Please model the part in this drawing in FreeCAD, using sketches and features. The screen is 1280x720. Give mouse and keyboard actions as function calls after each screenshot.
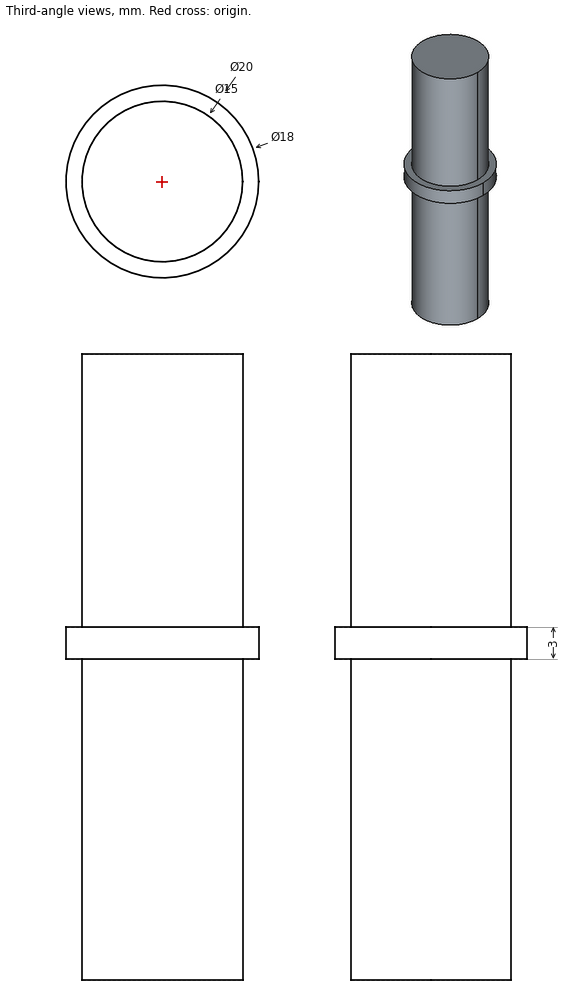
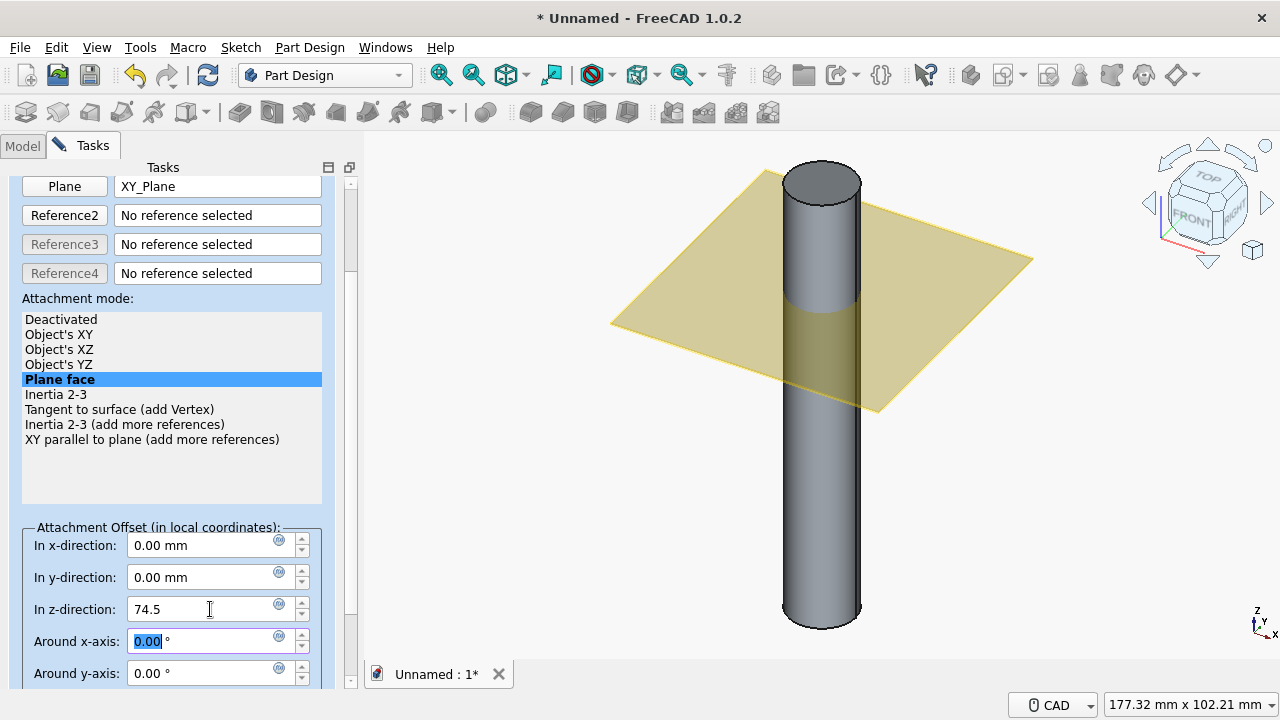
scroll(351, 432, up, 3)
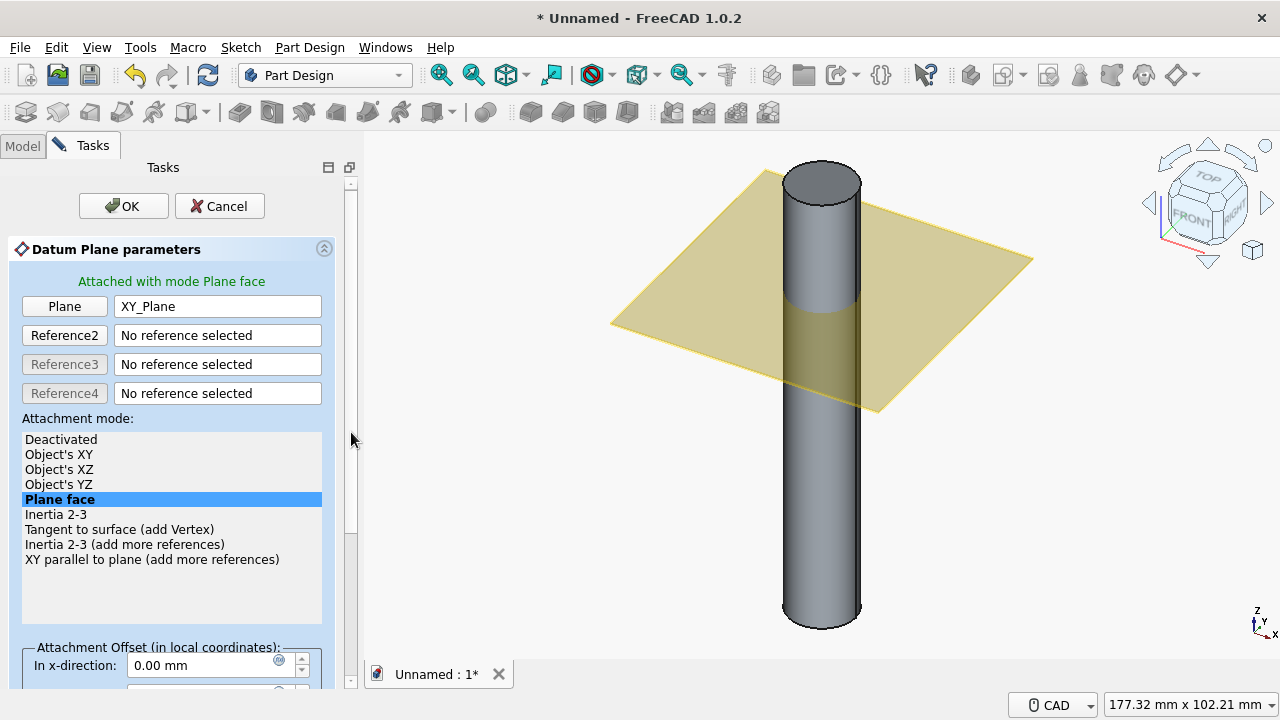
click(124, 206)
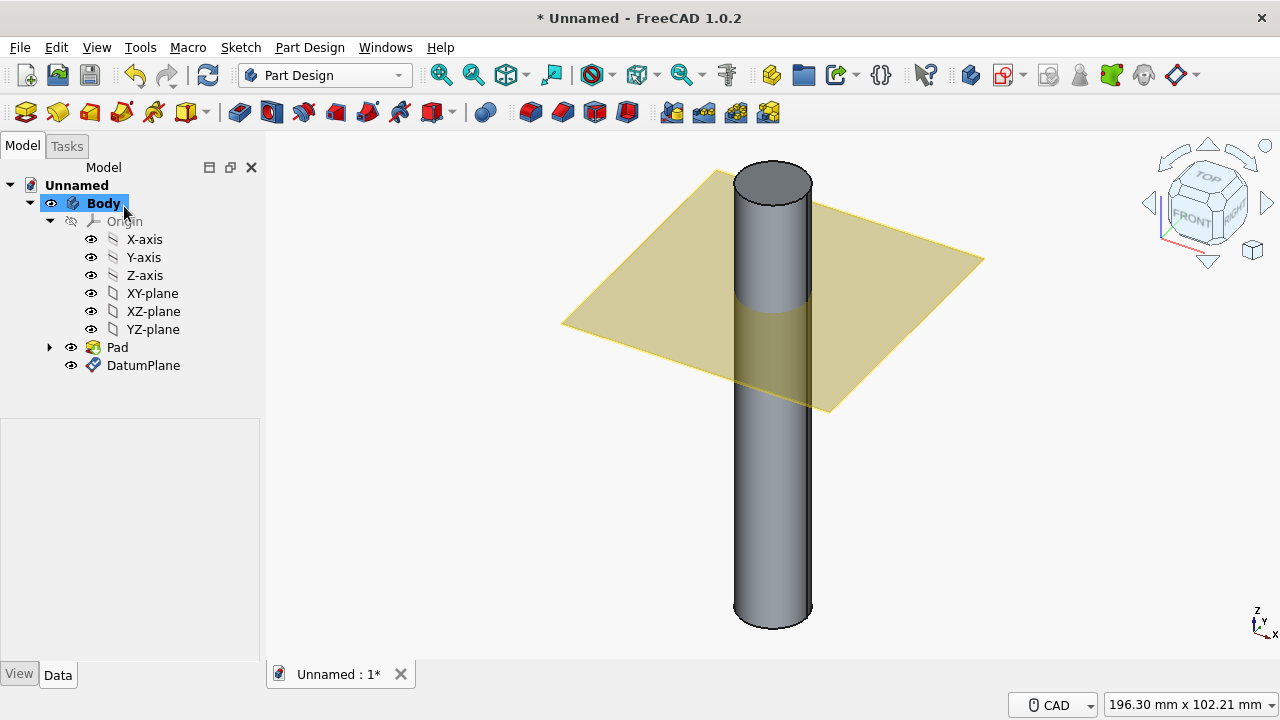
click(116, 365)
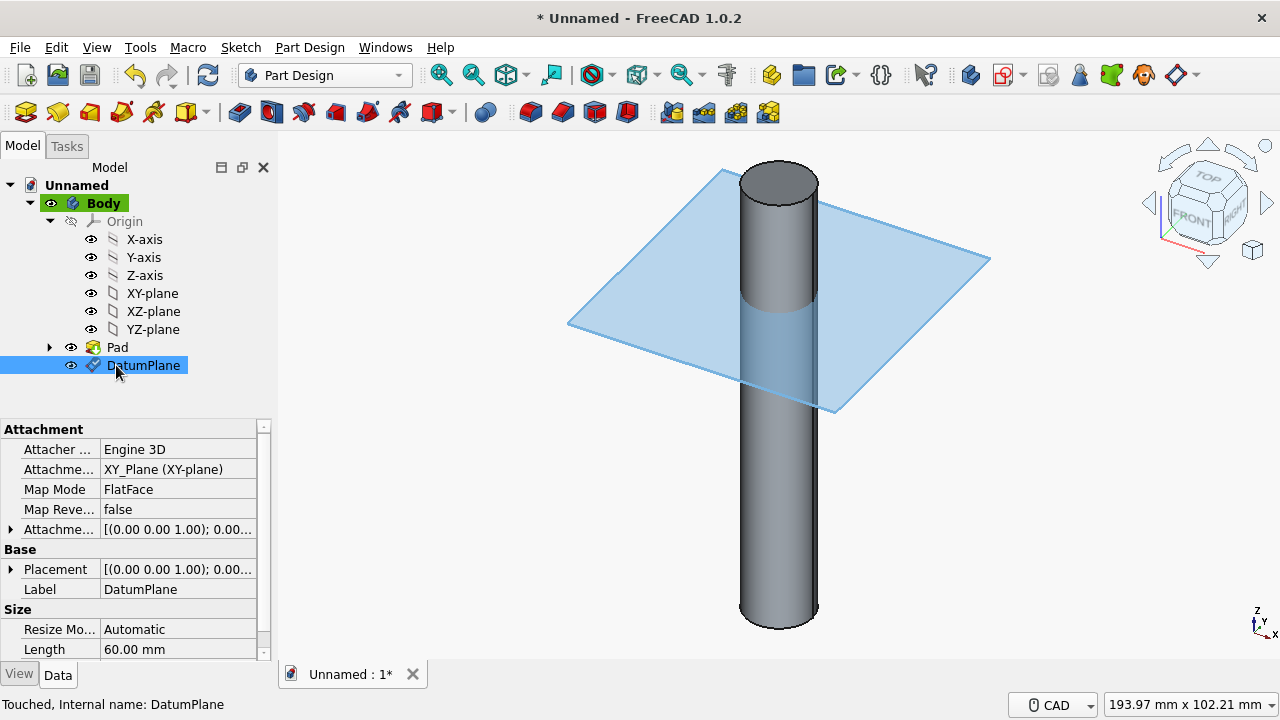
click(1004, 76)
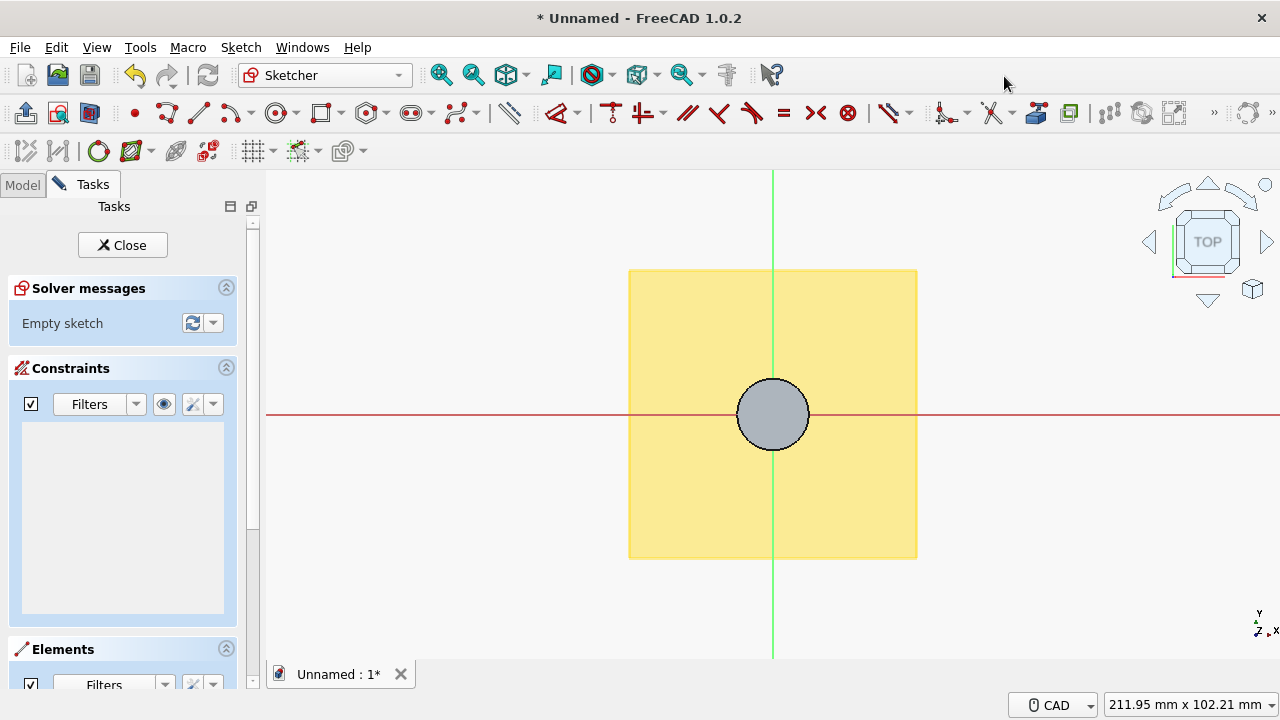
click(90, 114)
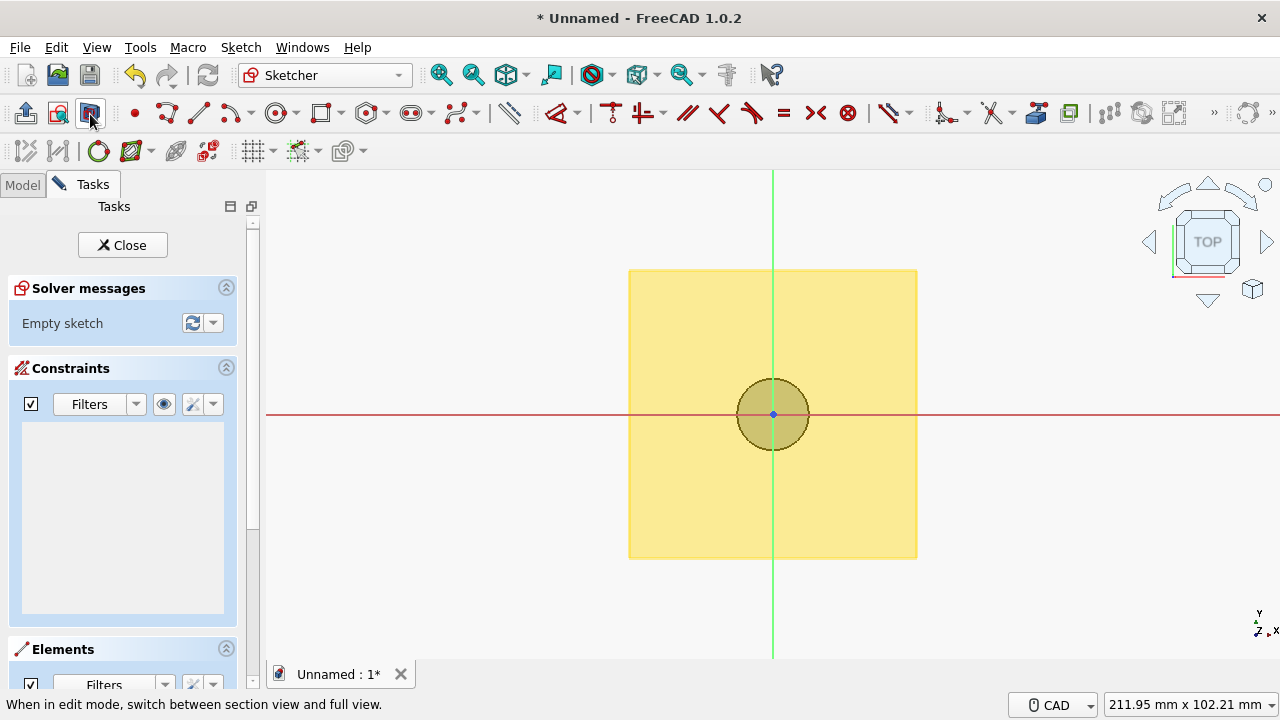
scroll(803, 415, up, 6)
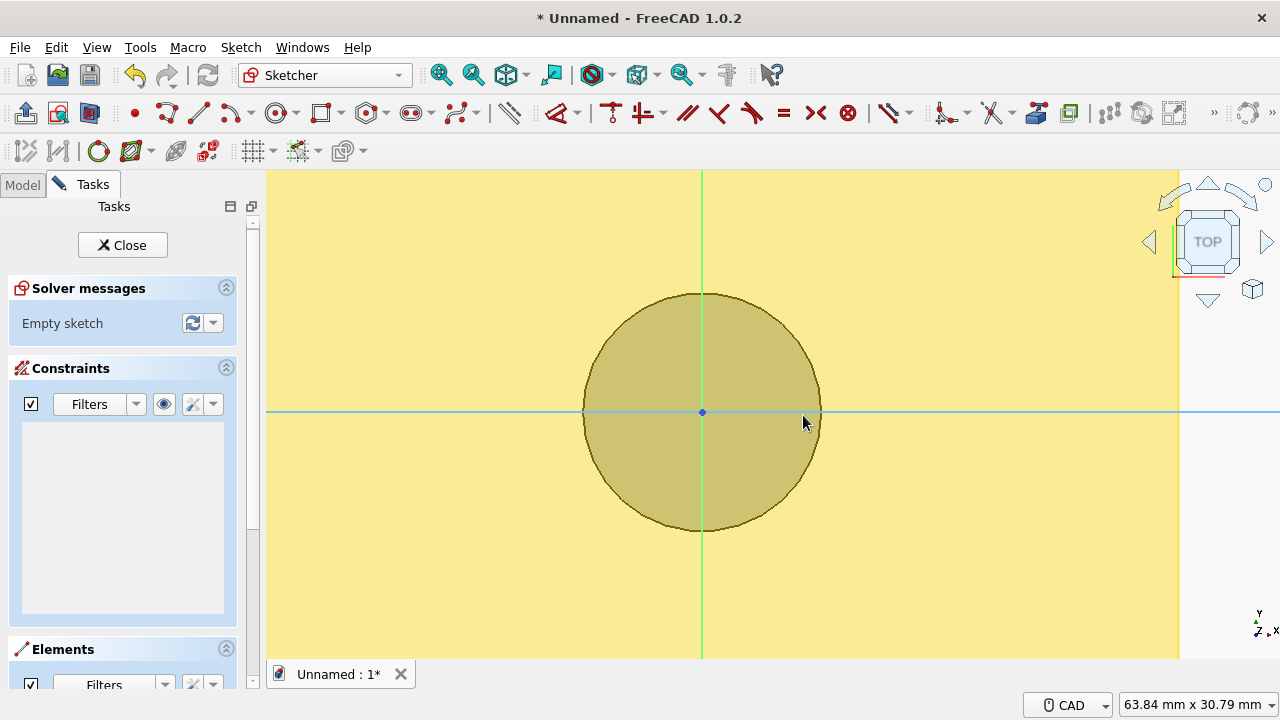
click(276, 114)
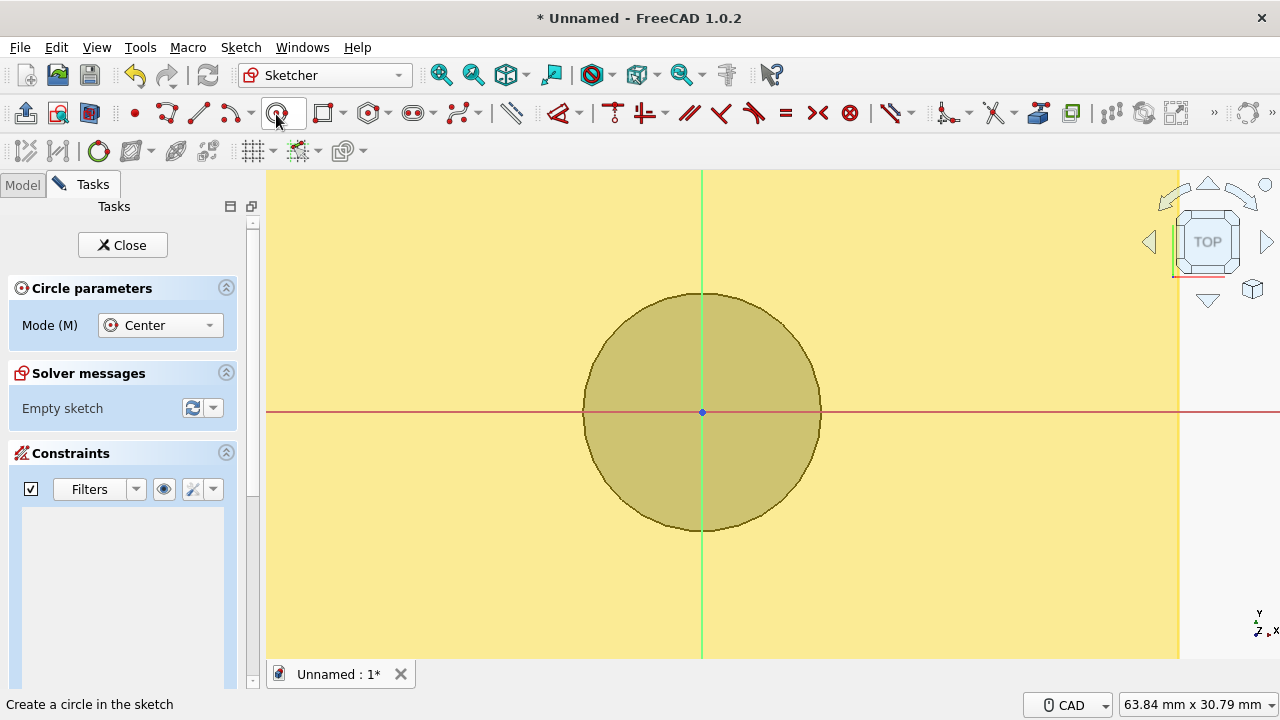
click(702, 412)
click(803, 311)
key(Escape)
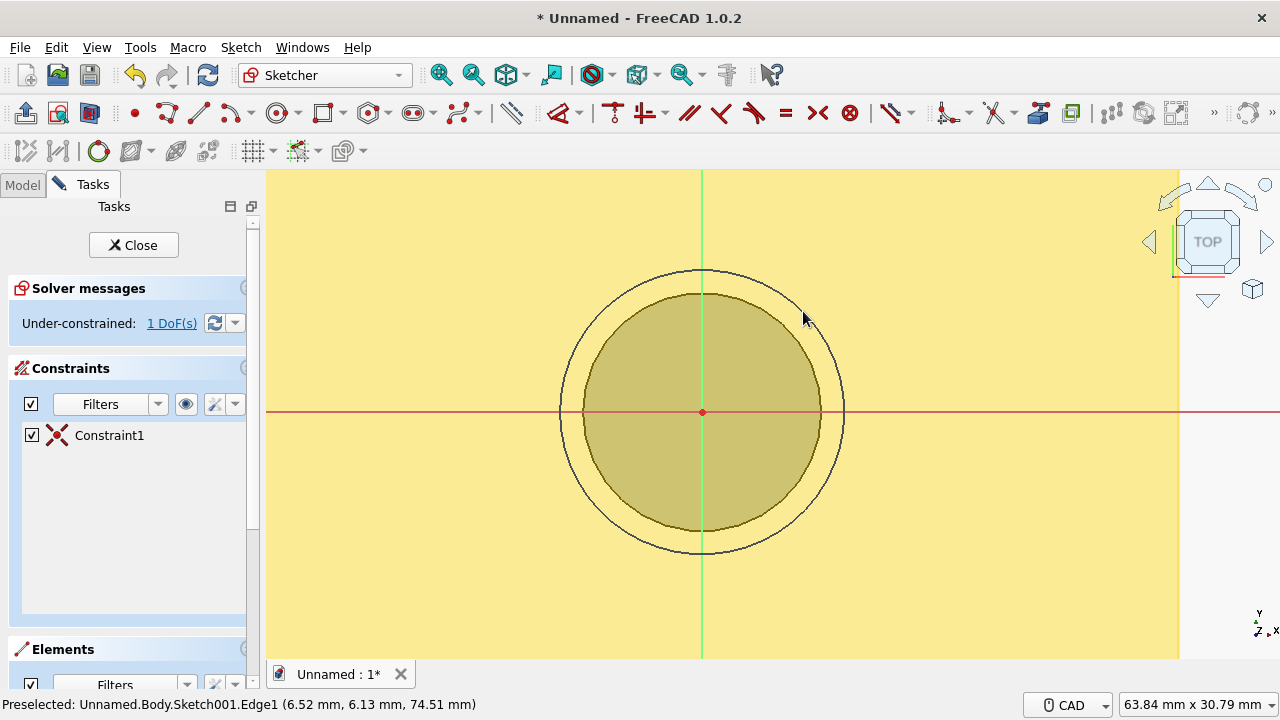
key(d)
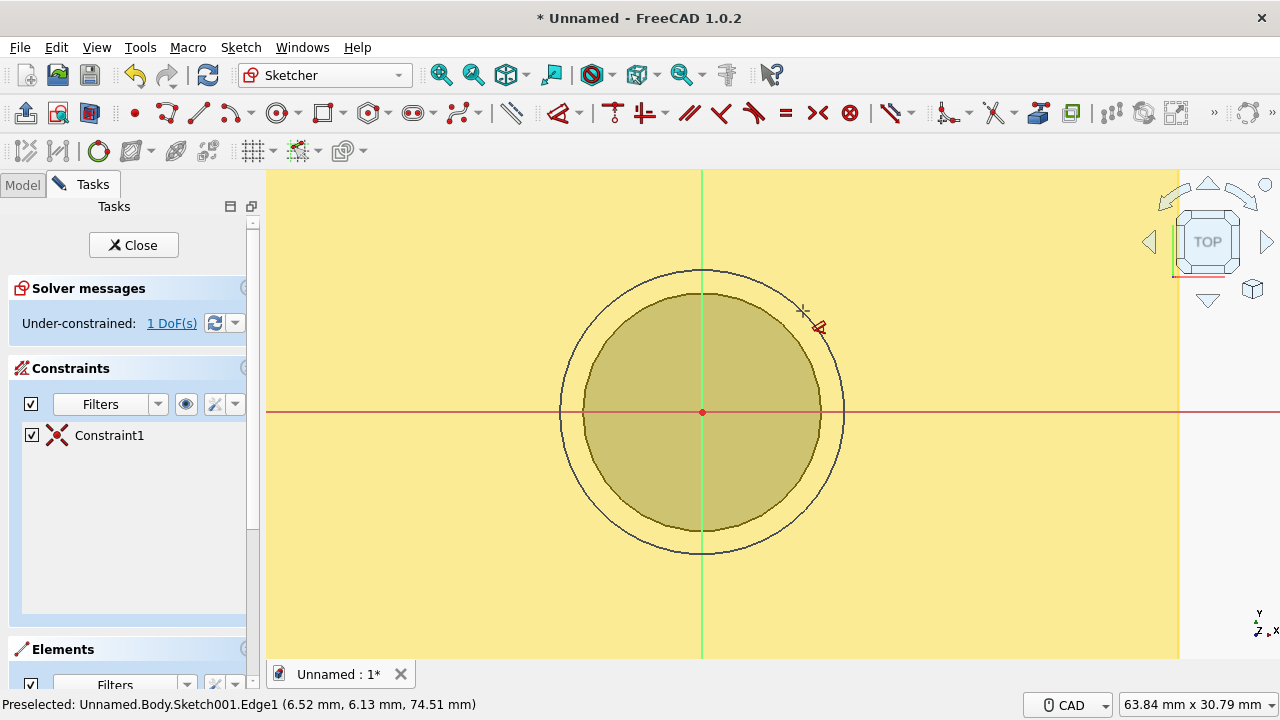
click(802, 311)
click(824, 288)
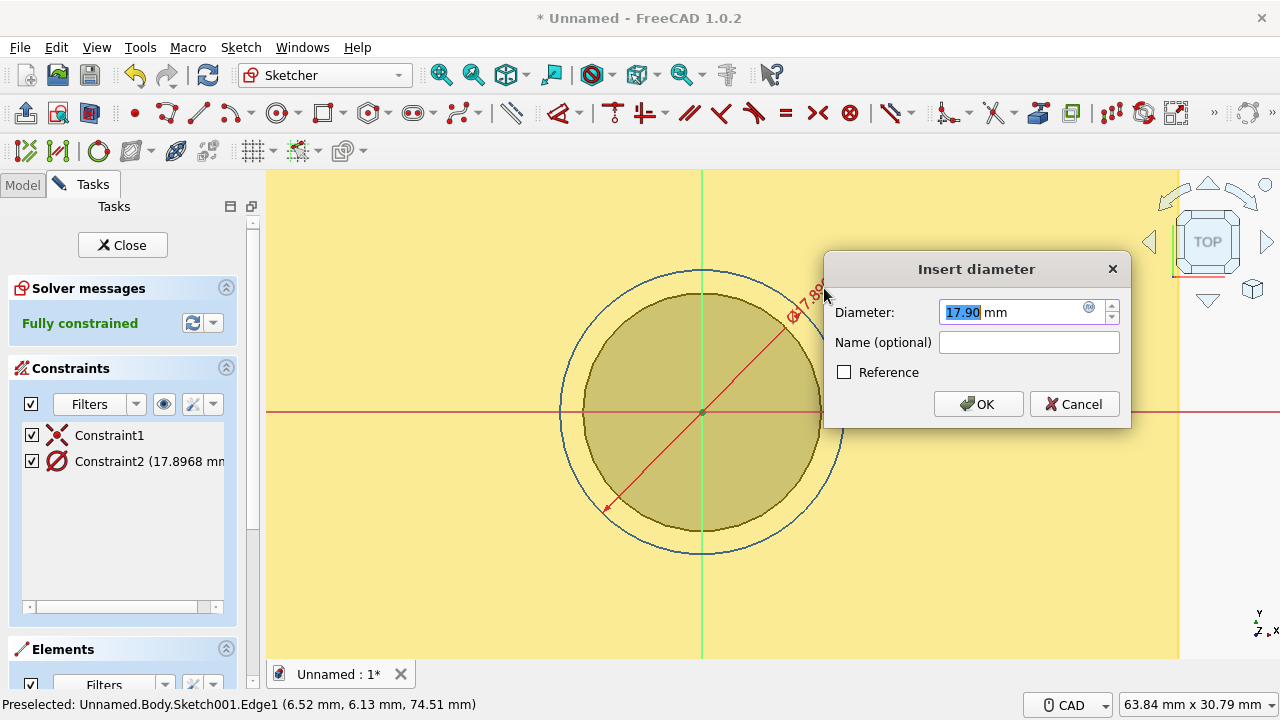
text(18)
key(Return)
key(Escape)